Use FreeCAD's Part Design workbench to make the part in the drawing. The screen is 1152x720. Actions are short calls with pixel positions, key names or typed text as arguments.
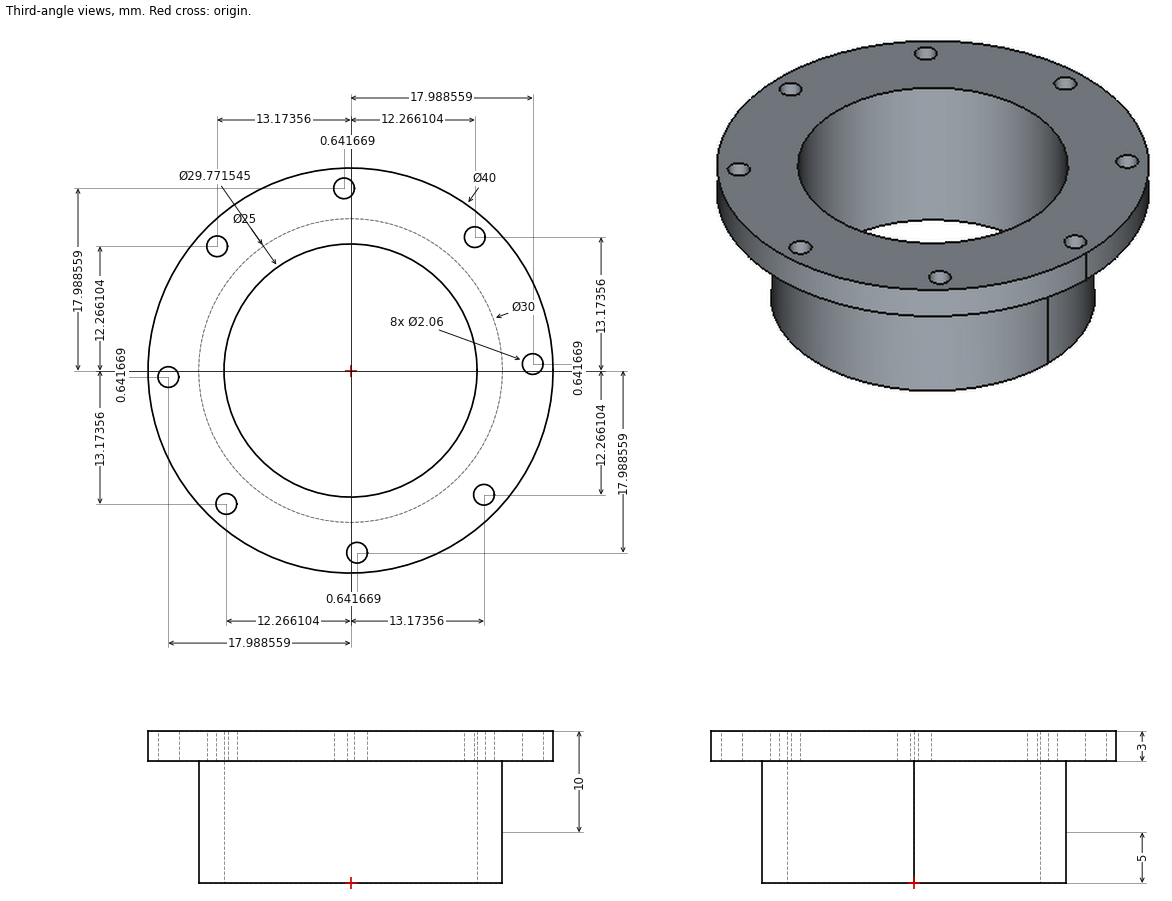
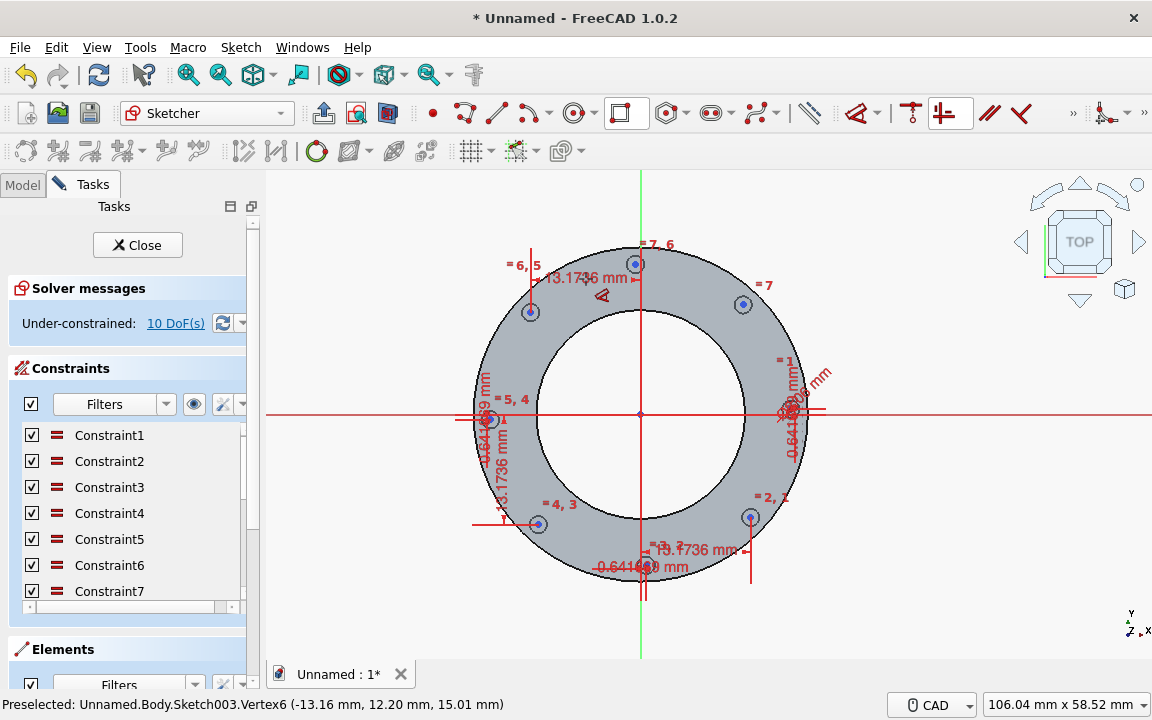
scroll(635, 264, up, 11)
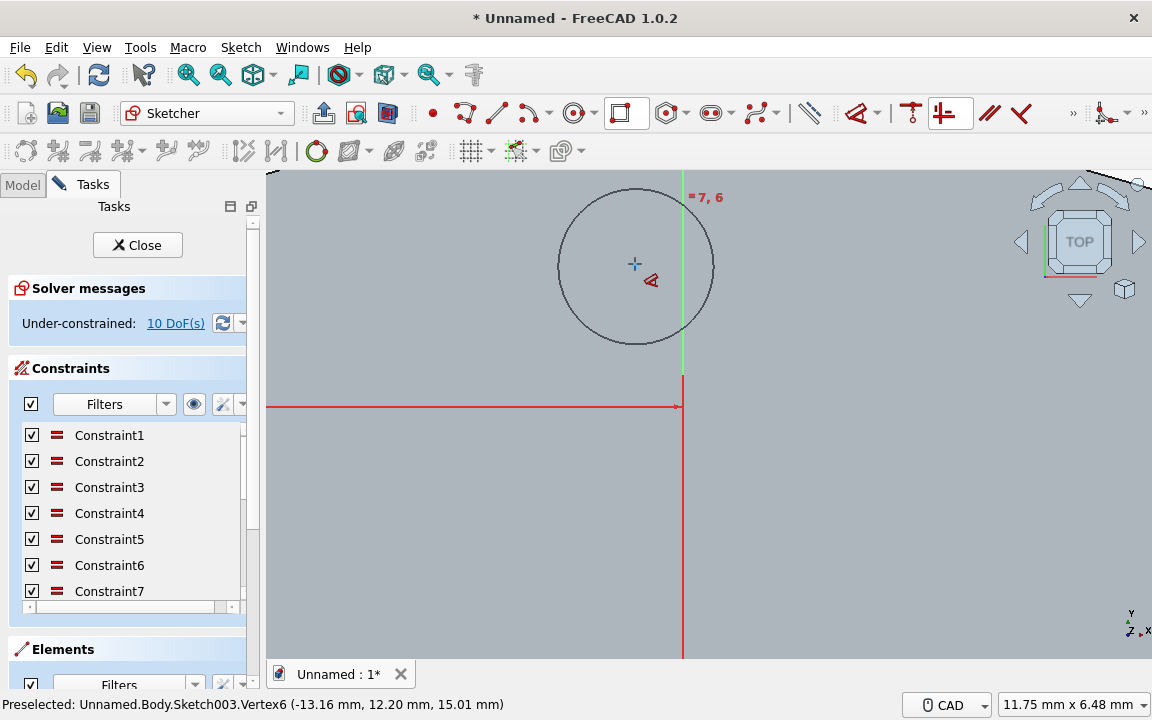
click(636, 267)
click(659, 233)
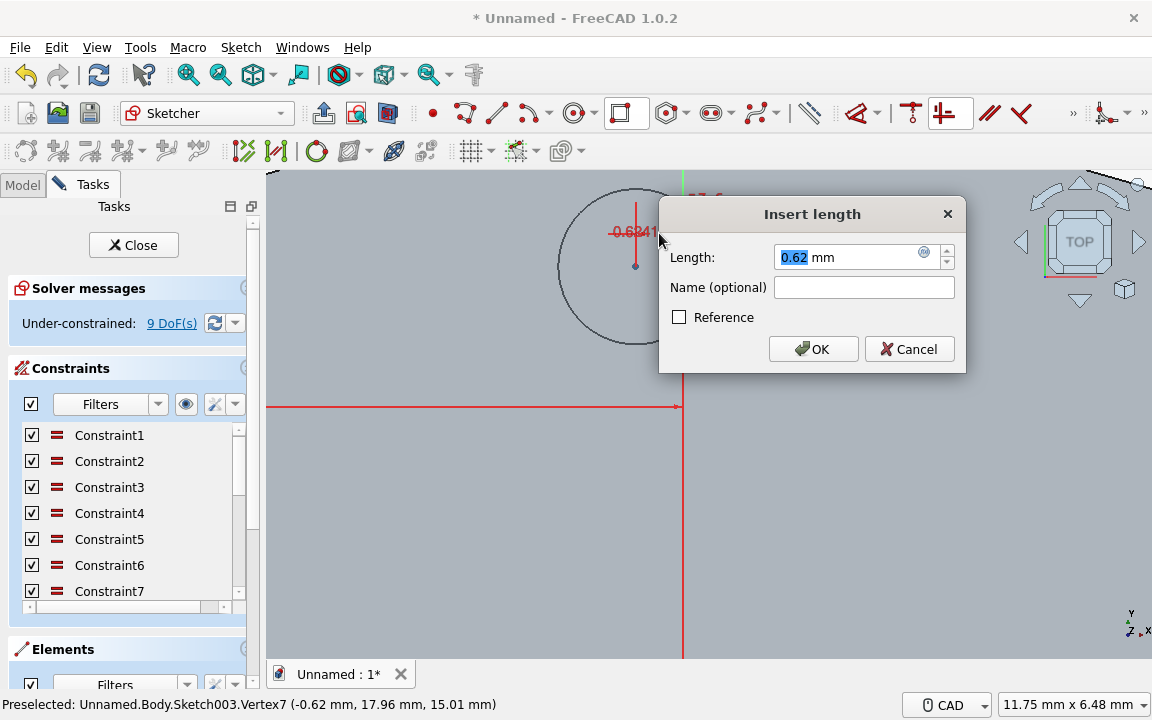
text(0.641669)
key(Return)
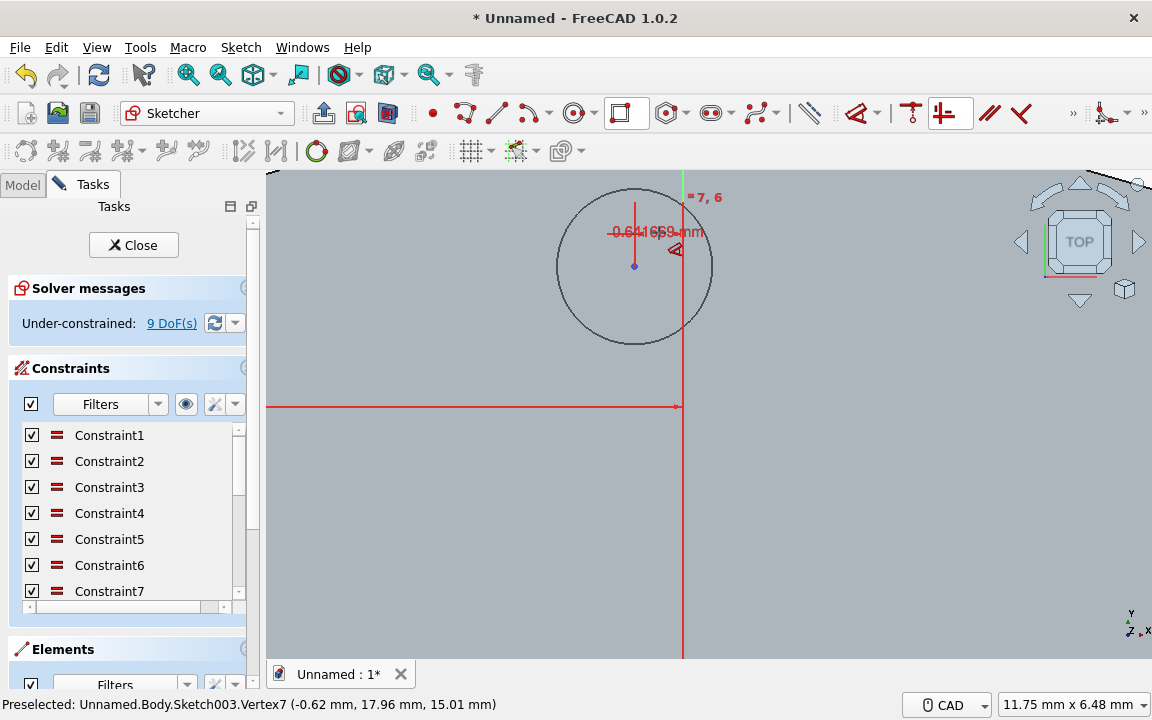
scroll(635, 264, down, 11)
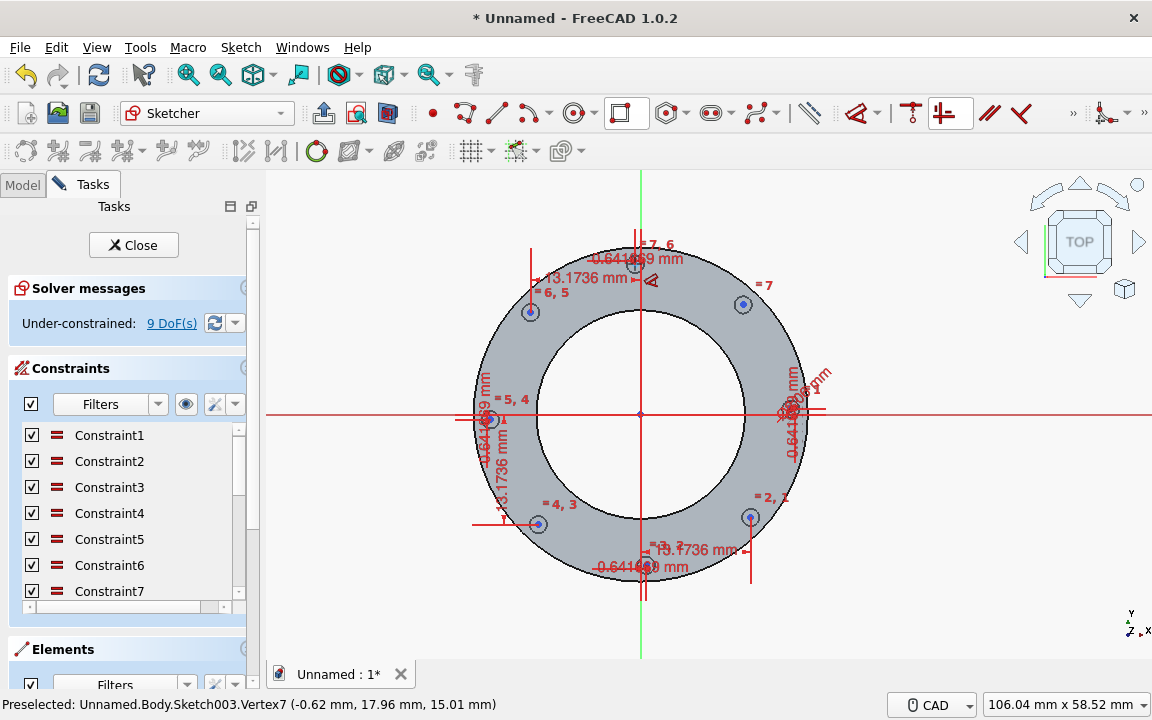
click(743, 305)
click(777, 360)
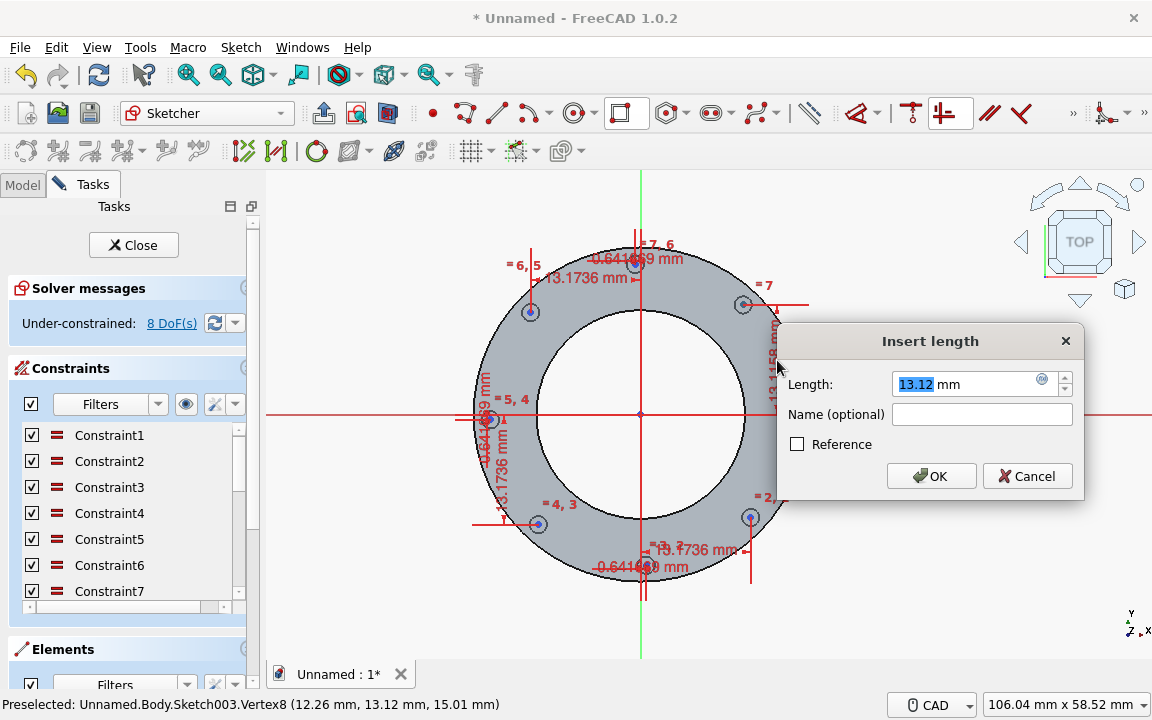
text(13.17356)
key(Return)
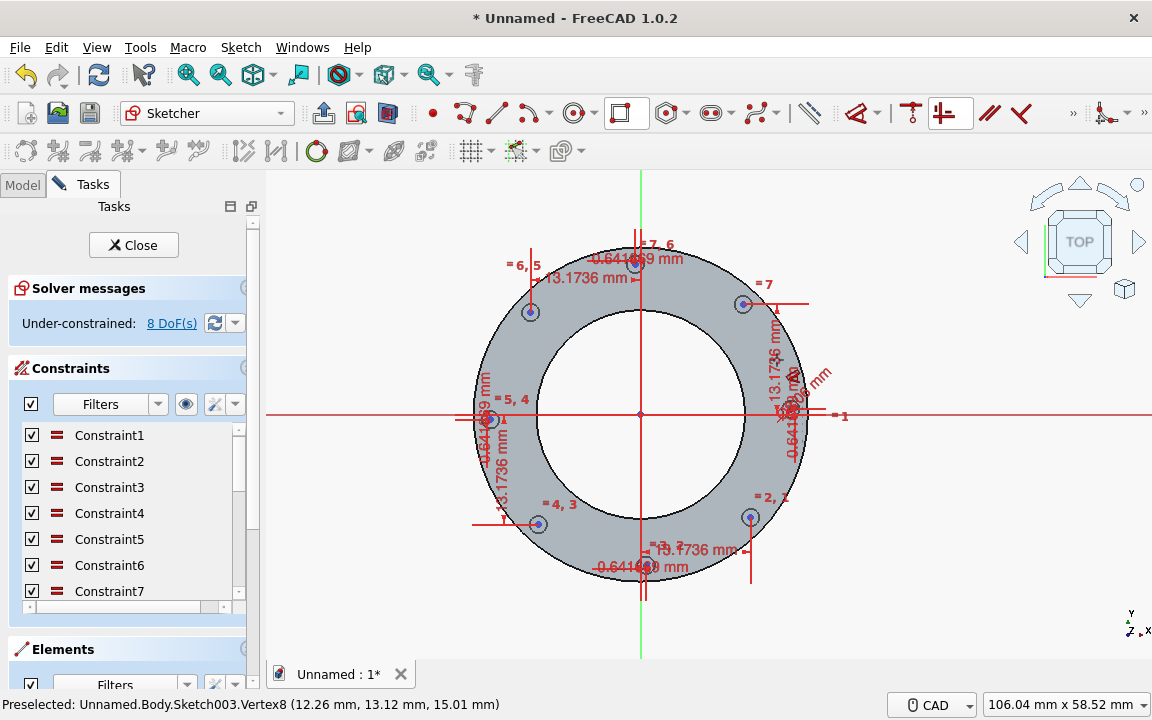
click(791, 409)
click(681, 375)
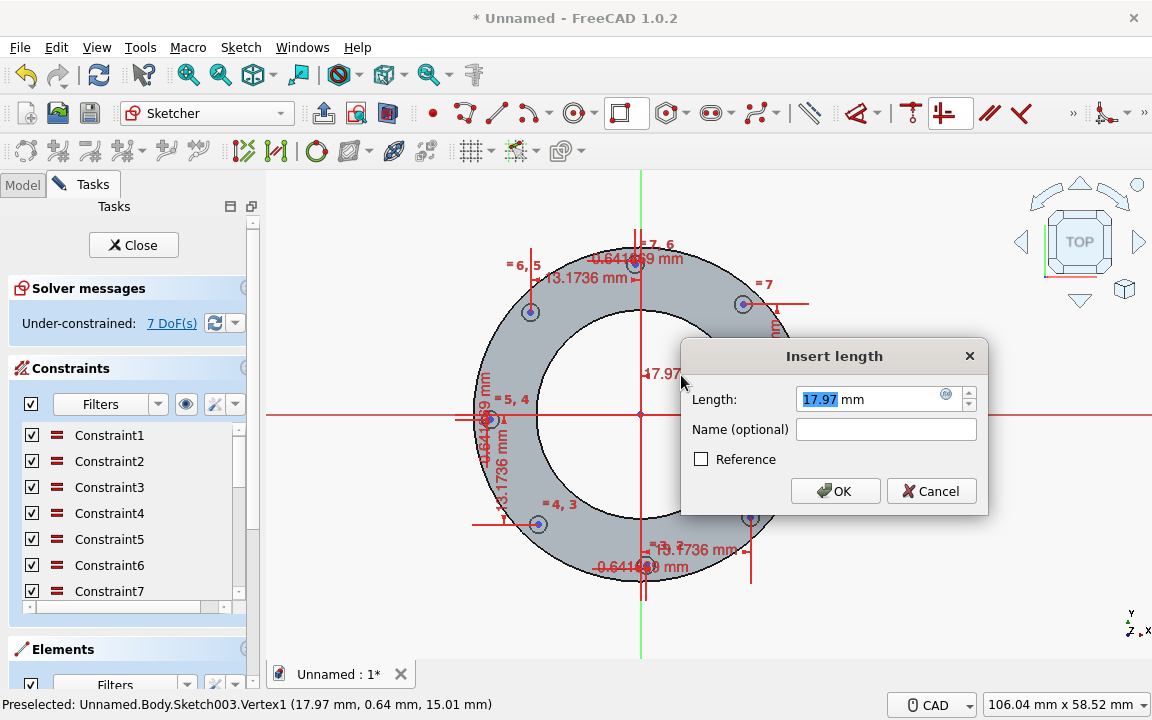
text(17.988559)
key(Return)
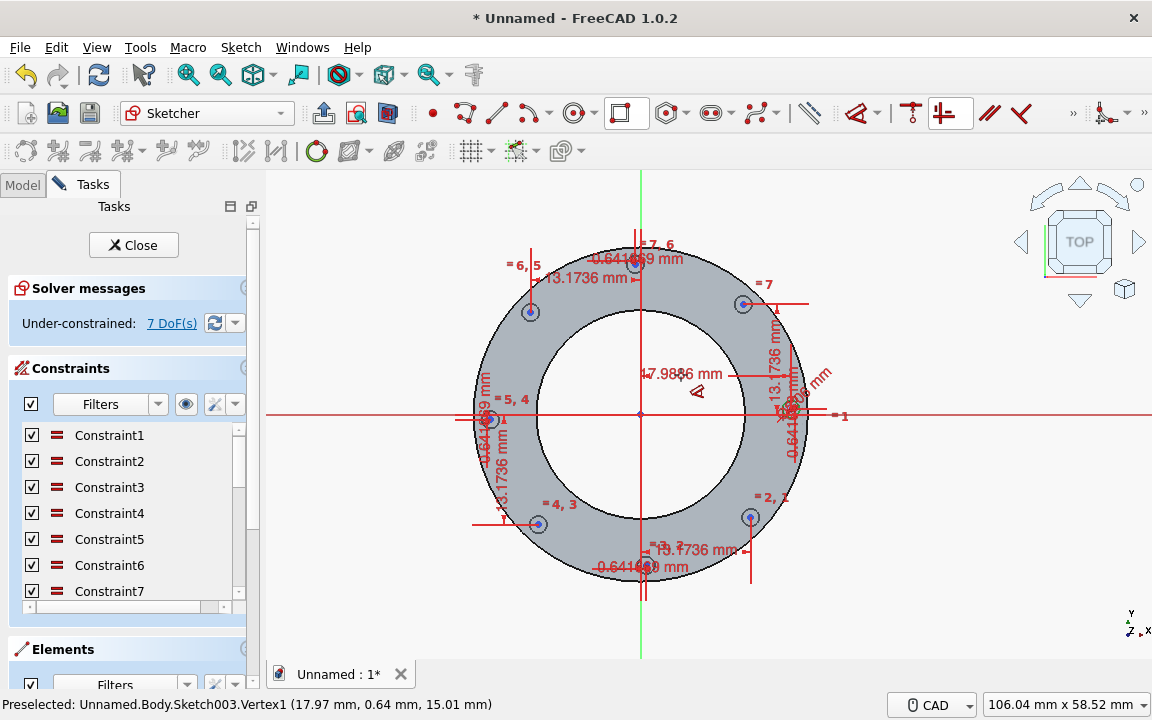
click(751, 517)
click(785, 466)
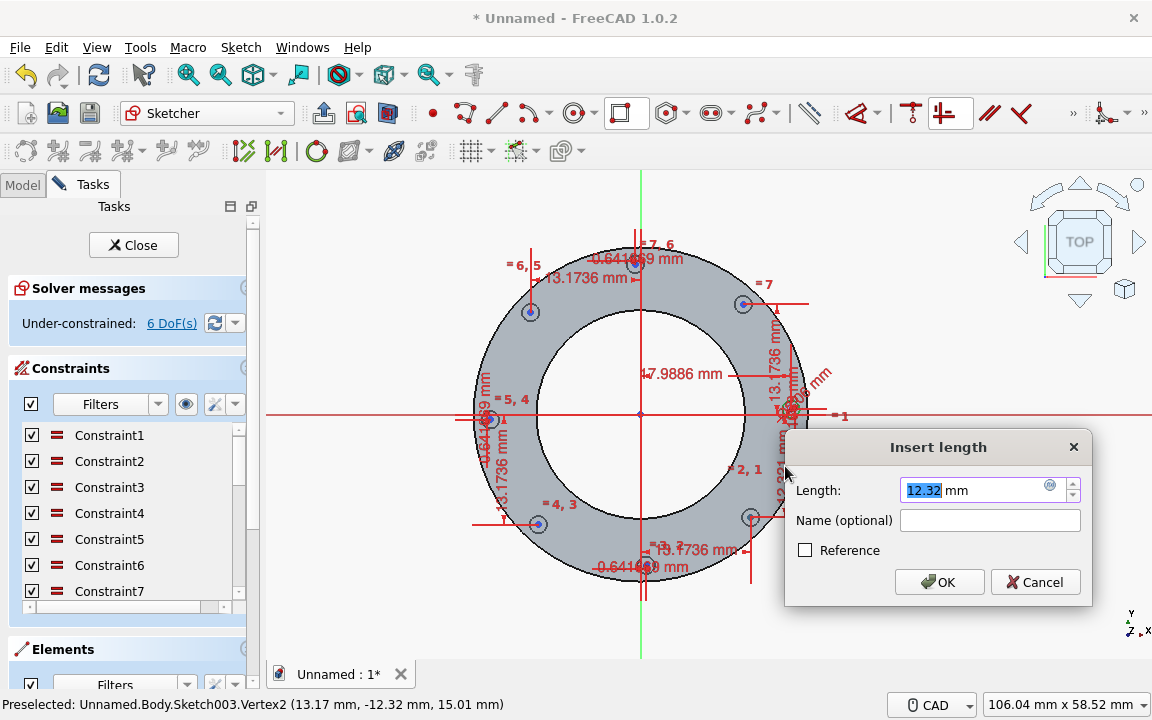
text(12.266104)
key(Return)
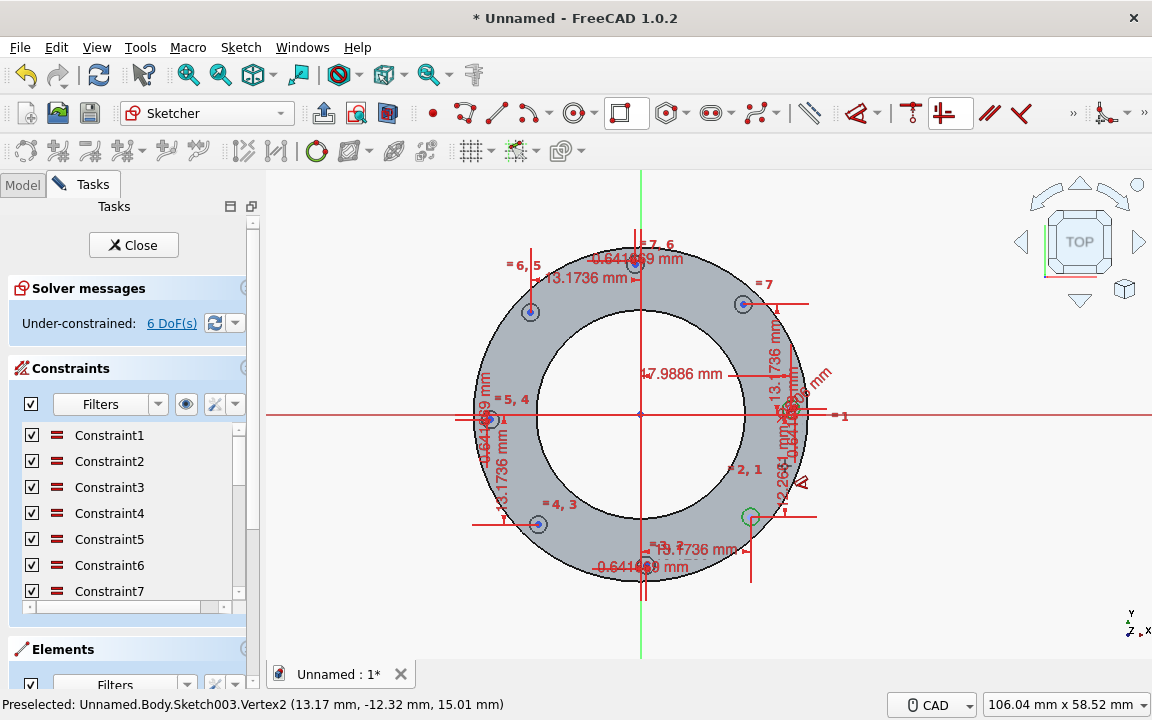
click(646, 565)
click(680, 490)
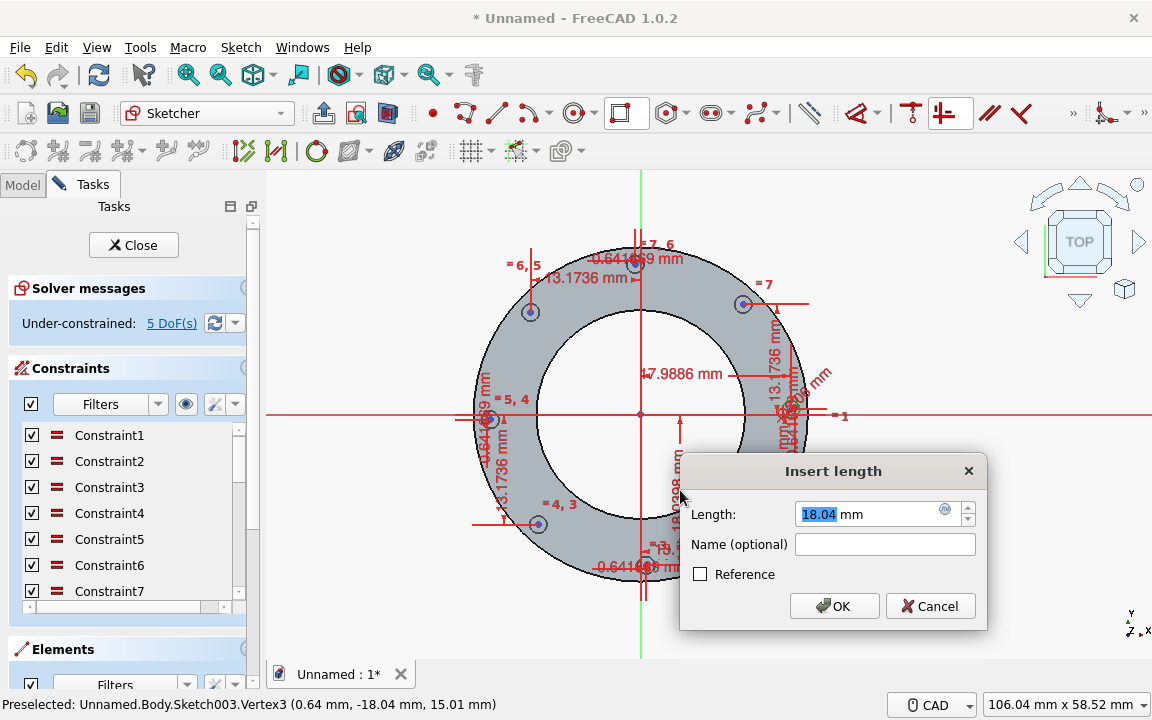
text(17.988559)
key(Return)